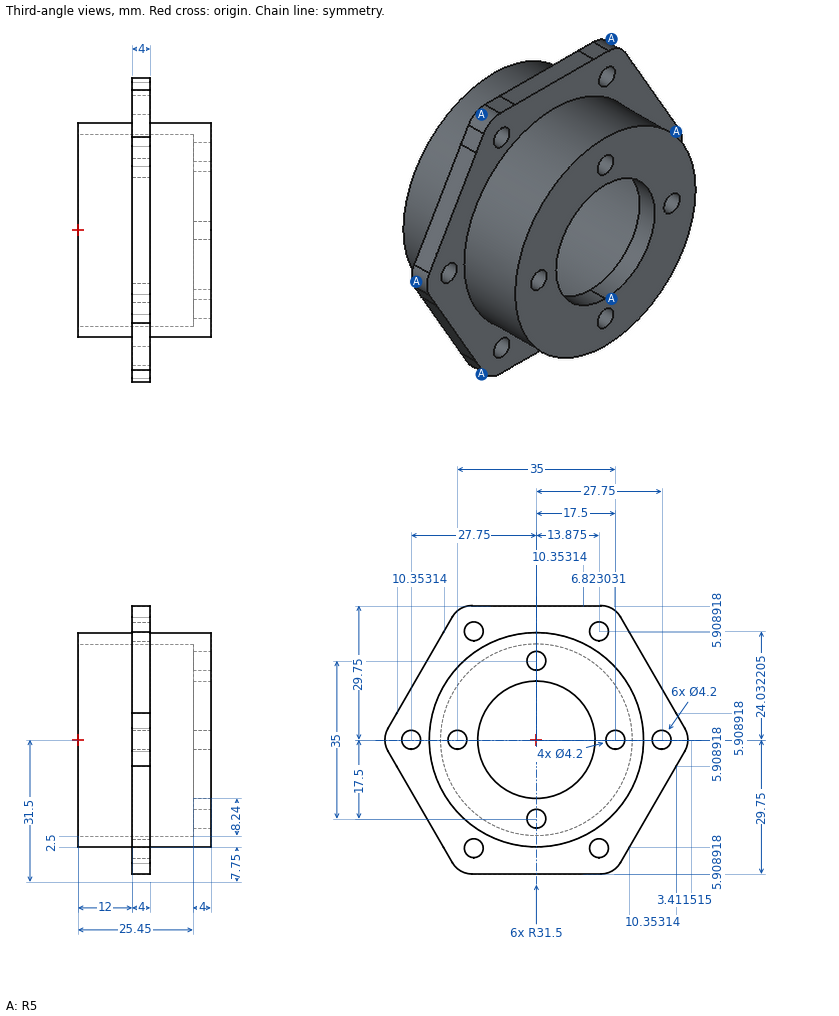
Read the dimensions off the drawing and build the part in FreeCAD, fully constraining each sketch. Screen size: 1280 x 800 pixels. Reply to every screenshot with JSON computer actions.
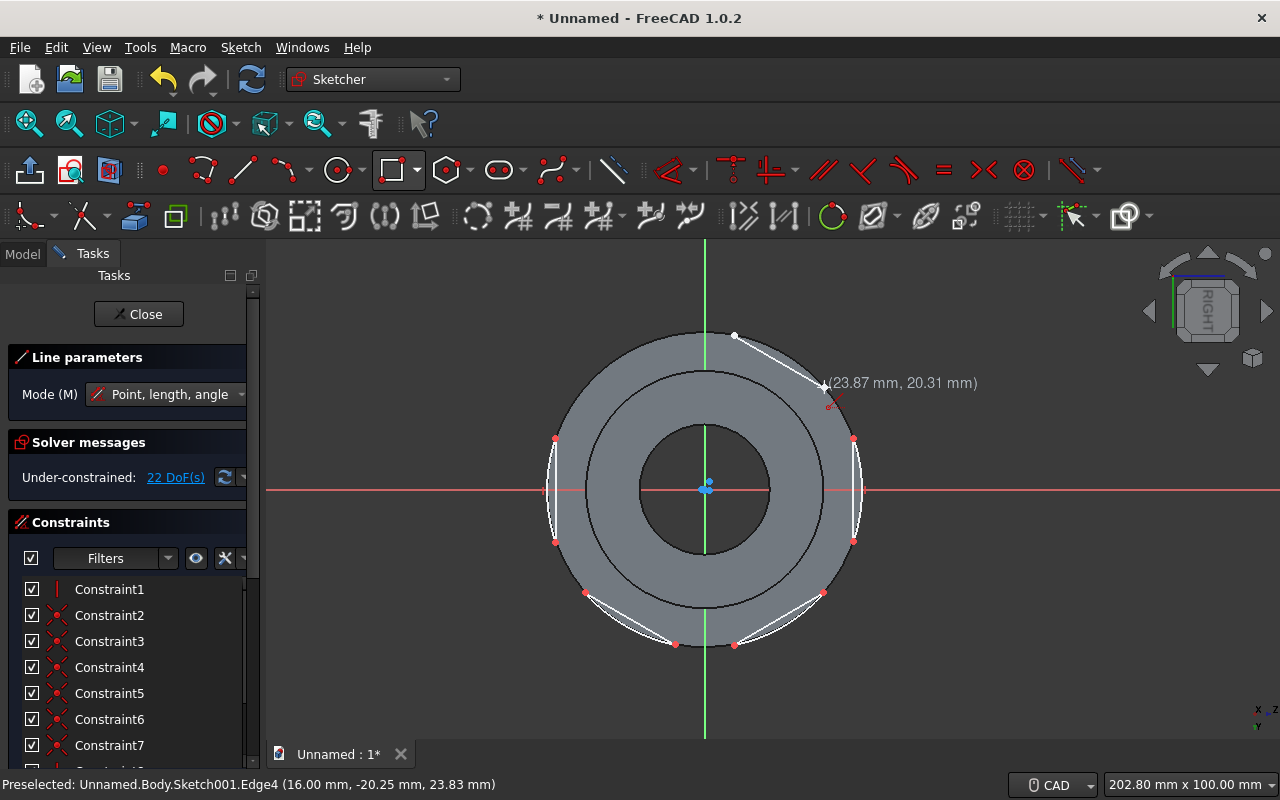
{"action": "key", "text": "g 3 a"}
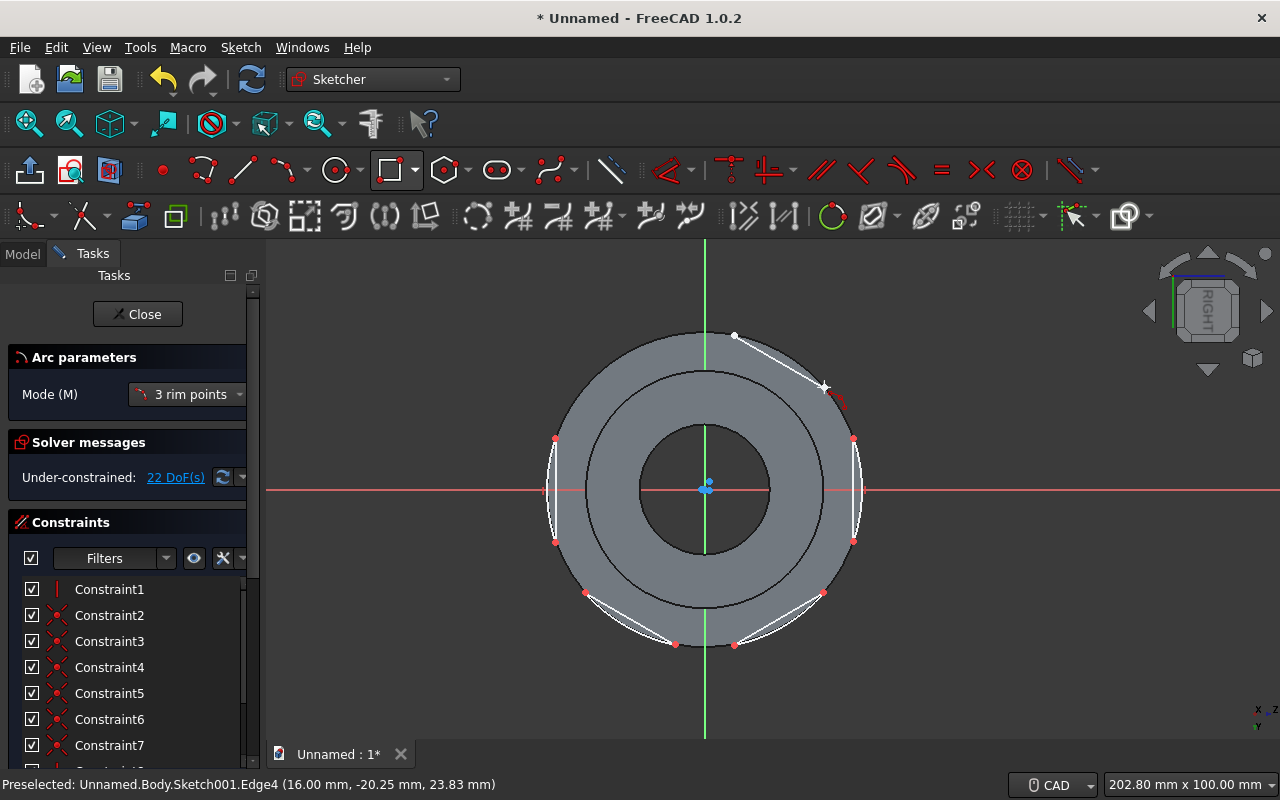
{"action": "left_click", "coordinate": [824, 388]}
{"action": "left_click", "coordinate": [734, 336]}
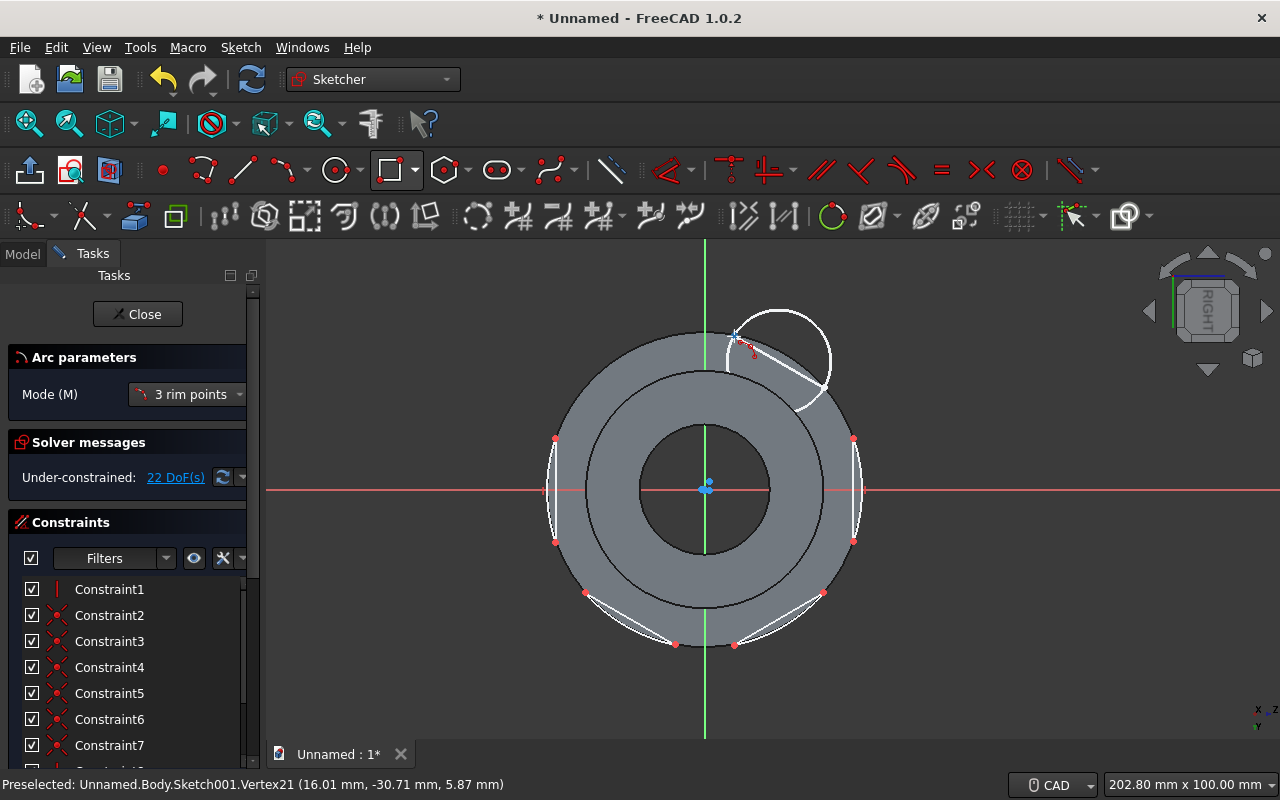
{"action": "scroll", "coordinate": [783, 353], "scroll_direction": "up", "scroll_amount": 3}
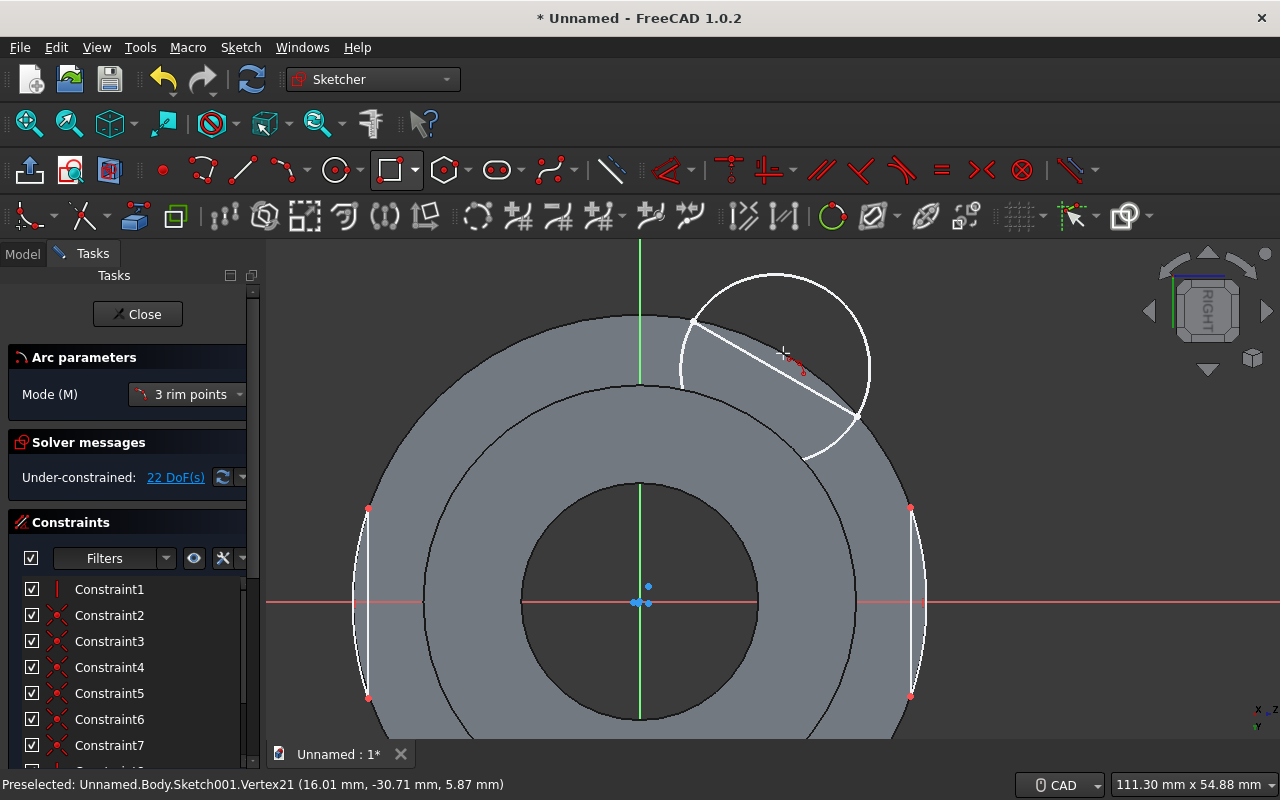
{"action": "left_click", "coordinate": [783, 353]}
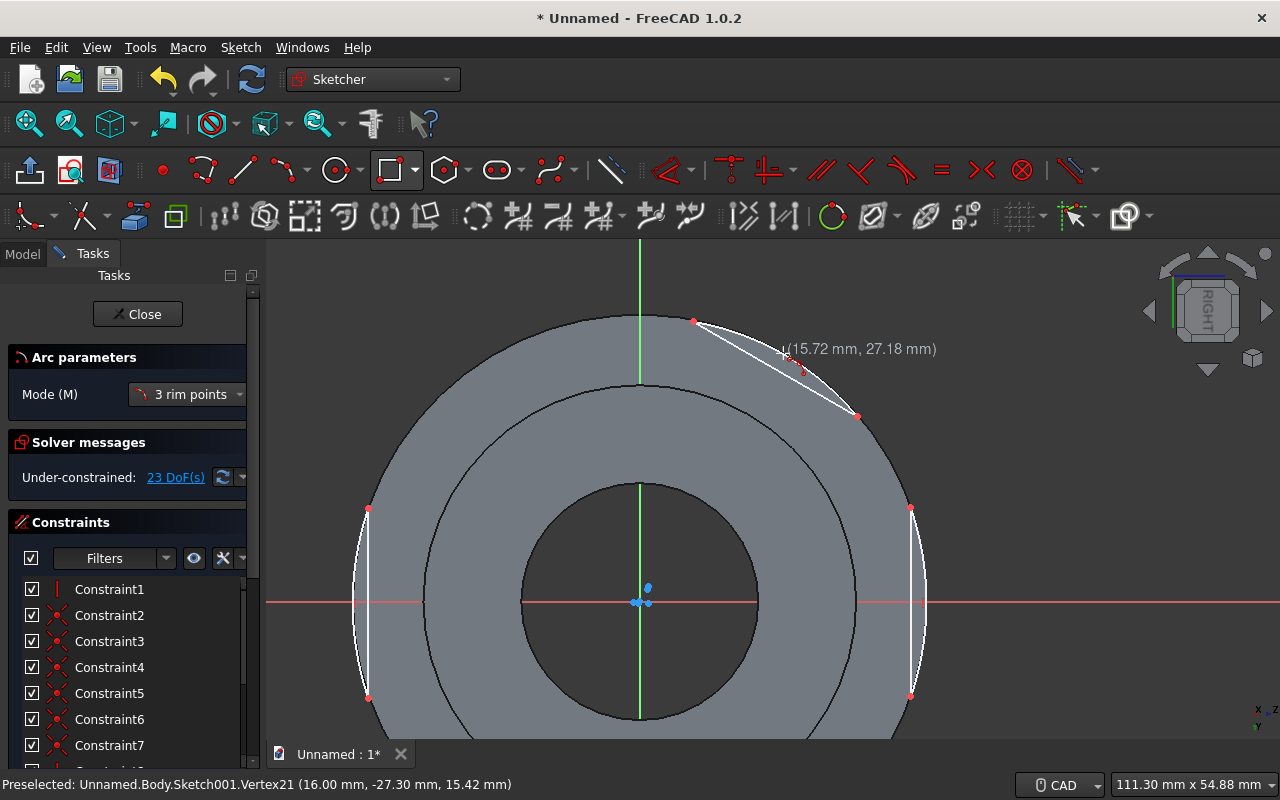
{"action": "key", "text": "g l"}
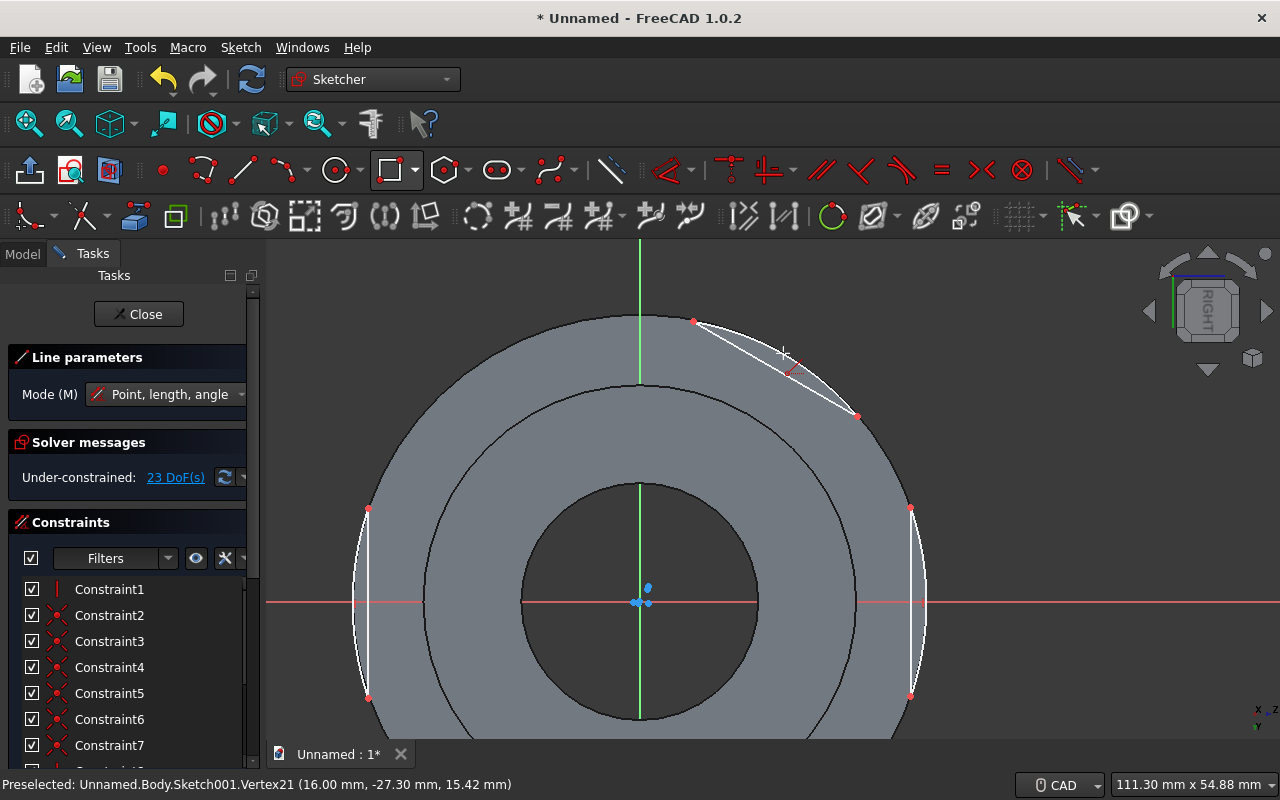
{"action": "left_click", "coordinate": [423, 414]}
{"action": "left_click", "coordinate": [586, 320]}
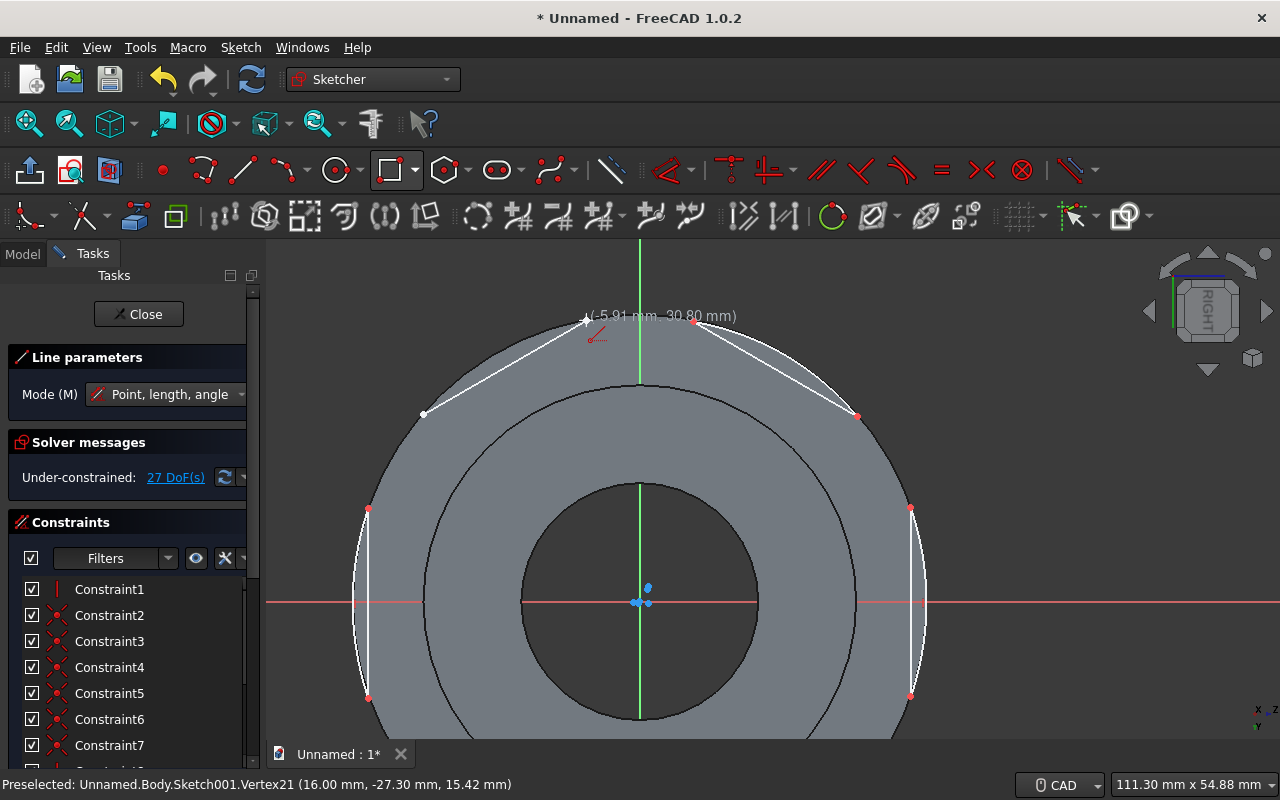
{"action": "left_click", "coordinate": [284, 170]}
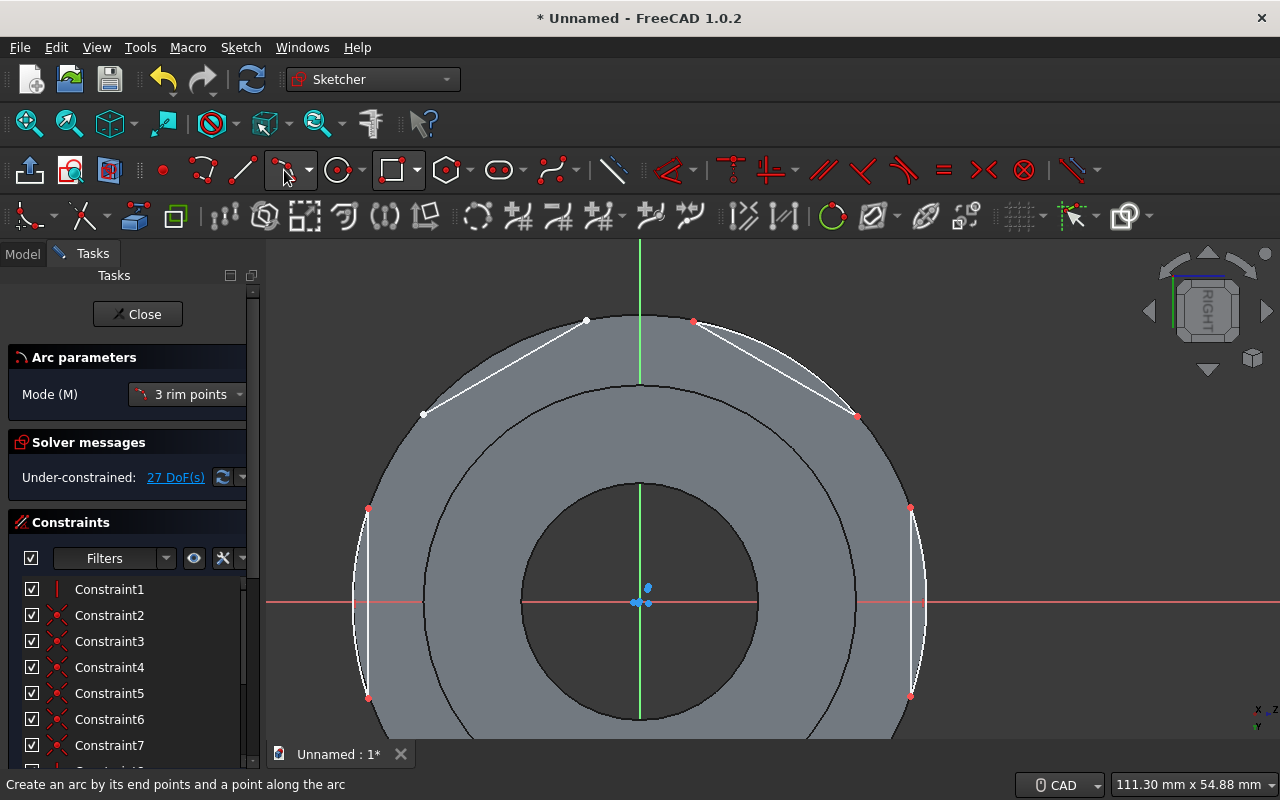
{"action": "left_click", "coordinate": [586, 321]}
{"action": "left_click", "coordinate": [423, 415]}
{"action": "left_click", "coordinate": [496, 353]}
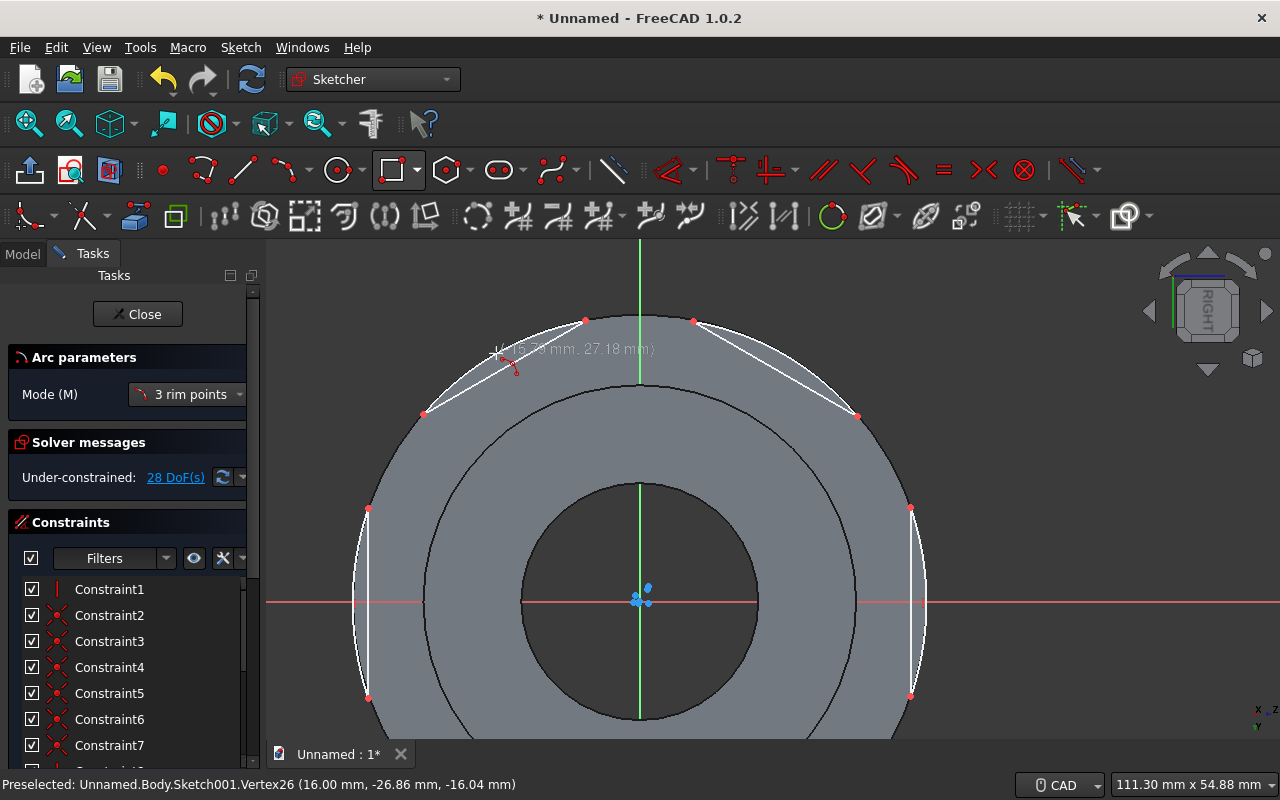
{"action": "key", "text": "g c"}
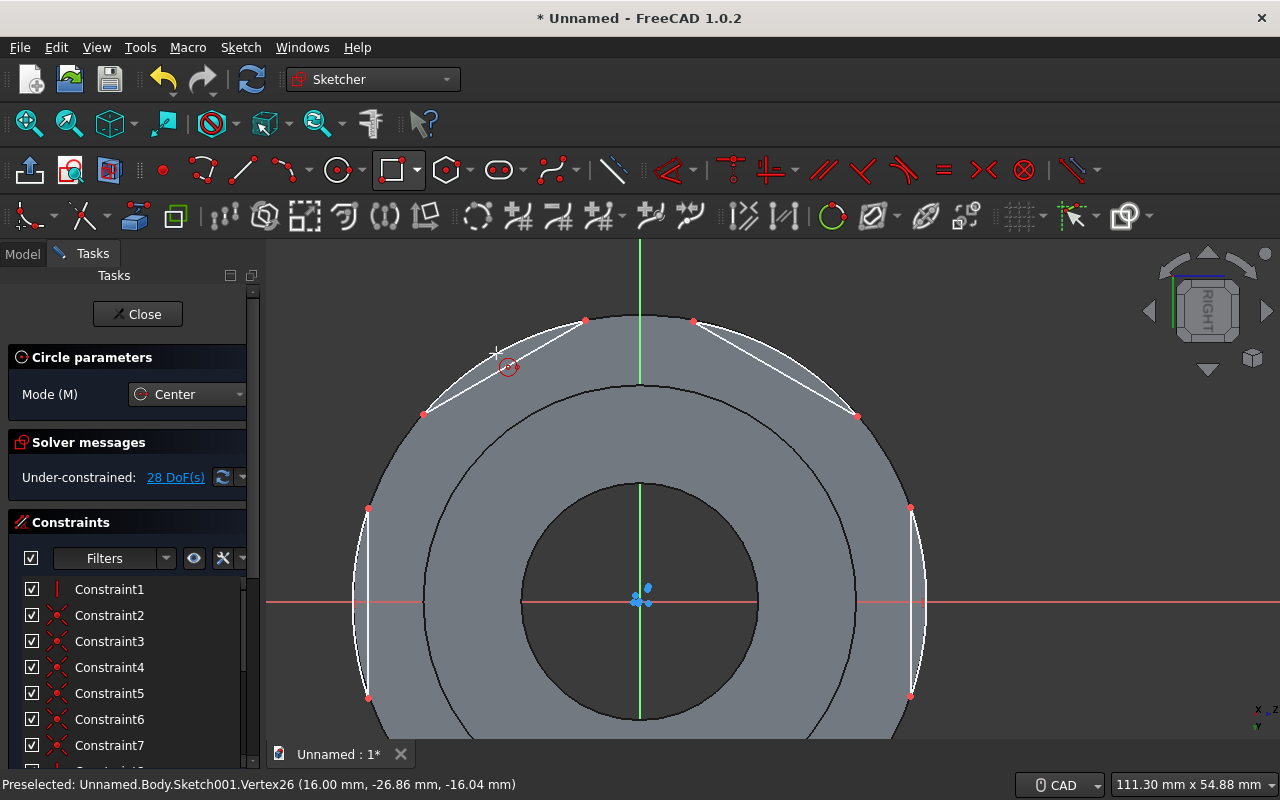
{"action": "scroll", "coordinate": [783, 352], "scroll_direction": "down", "scroll_amount": 3}